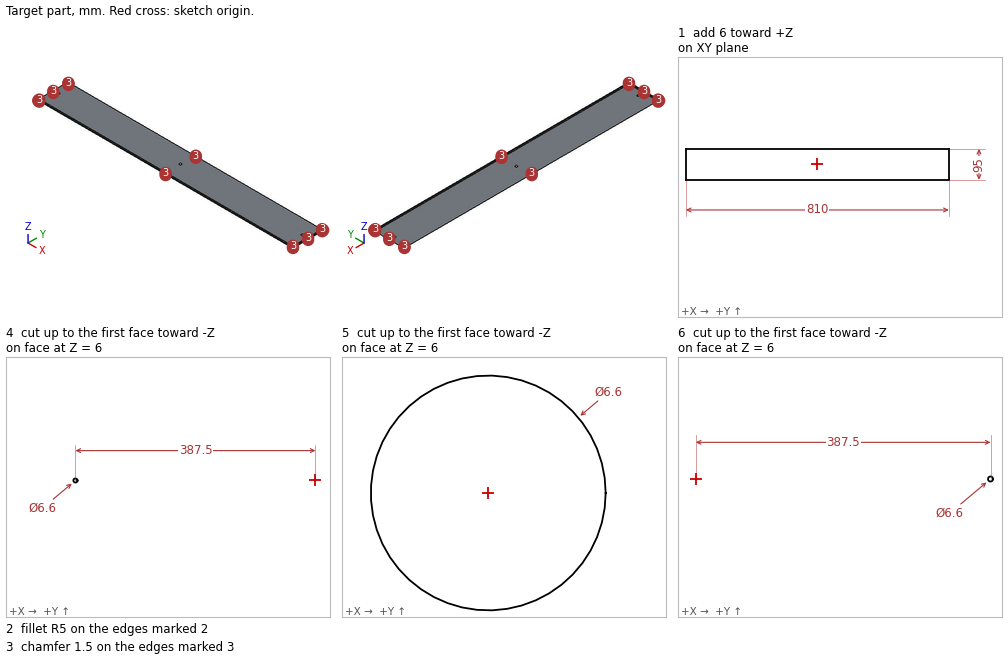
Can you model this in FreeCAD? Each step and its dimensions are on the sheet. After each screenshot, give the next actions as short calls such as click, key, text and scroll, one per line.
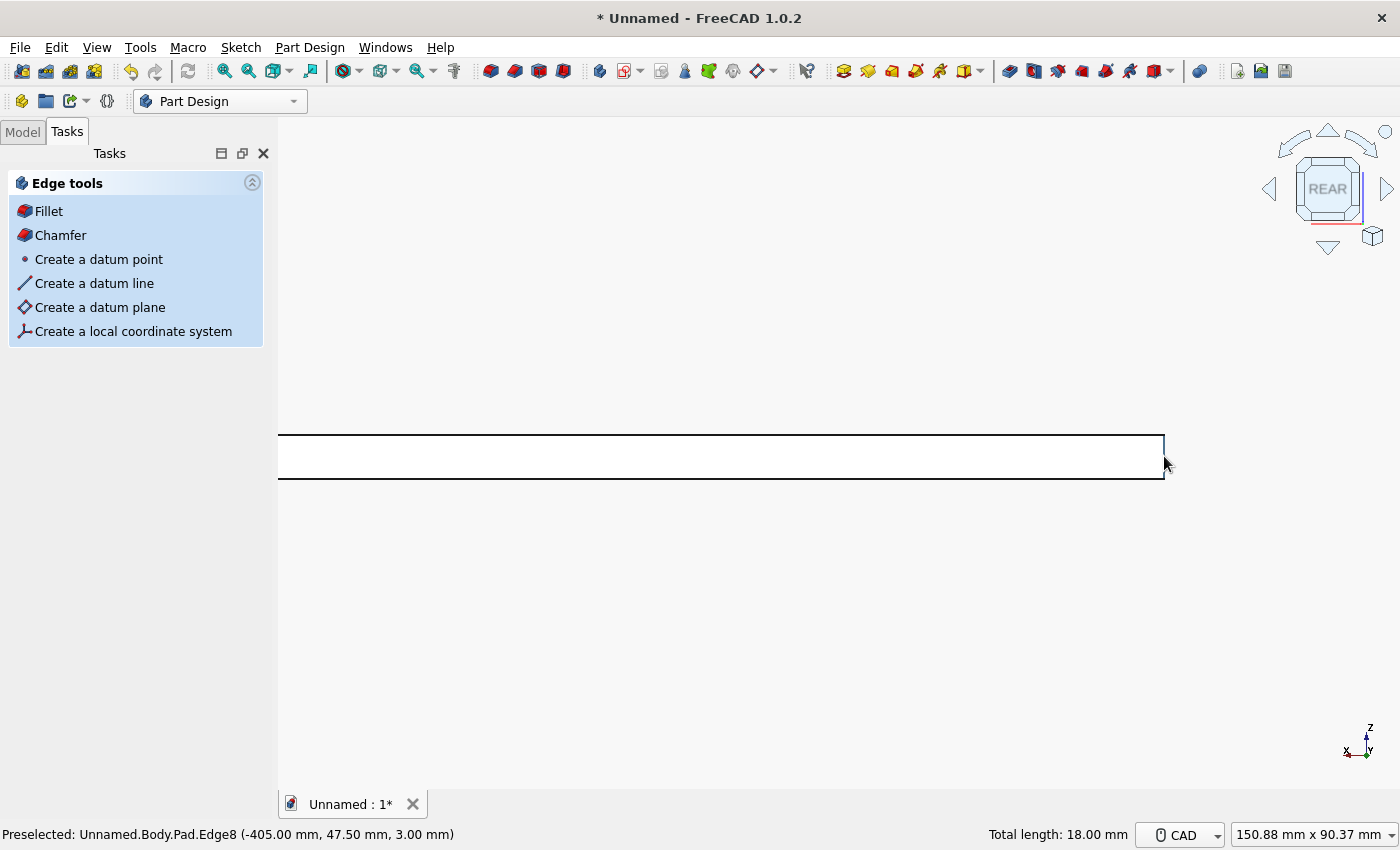
click(226, 72)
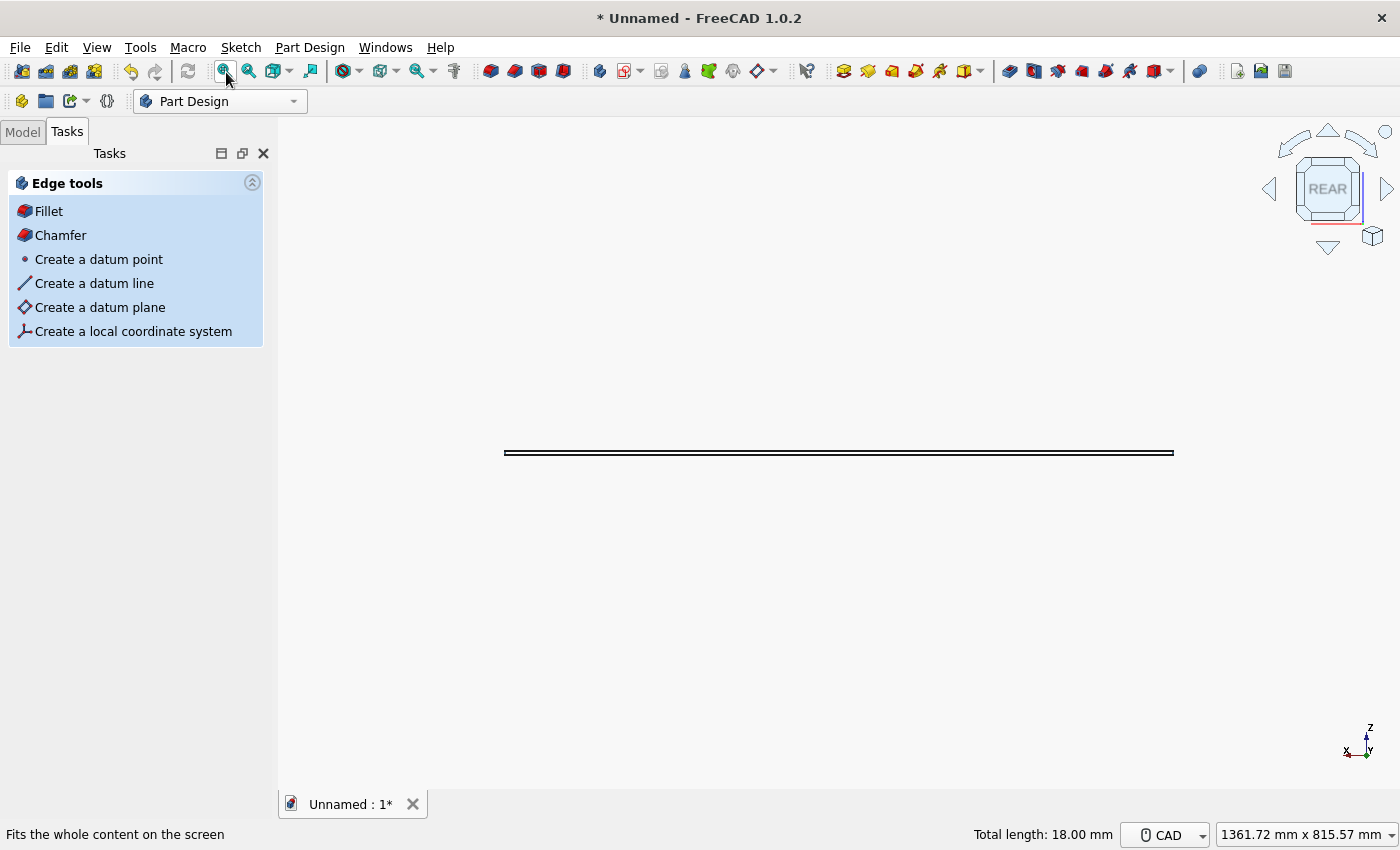
key(6)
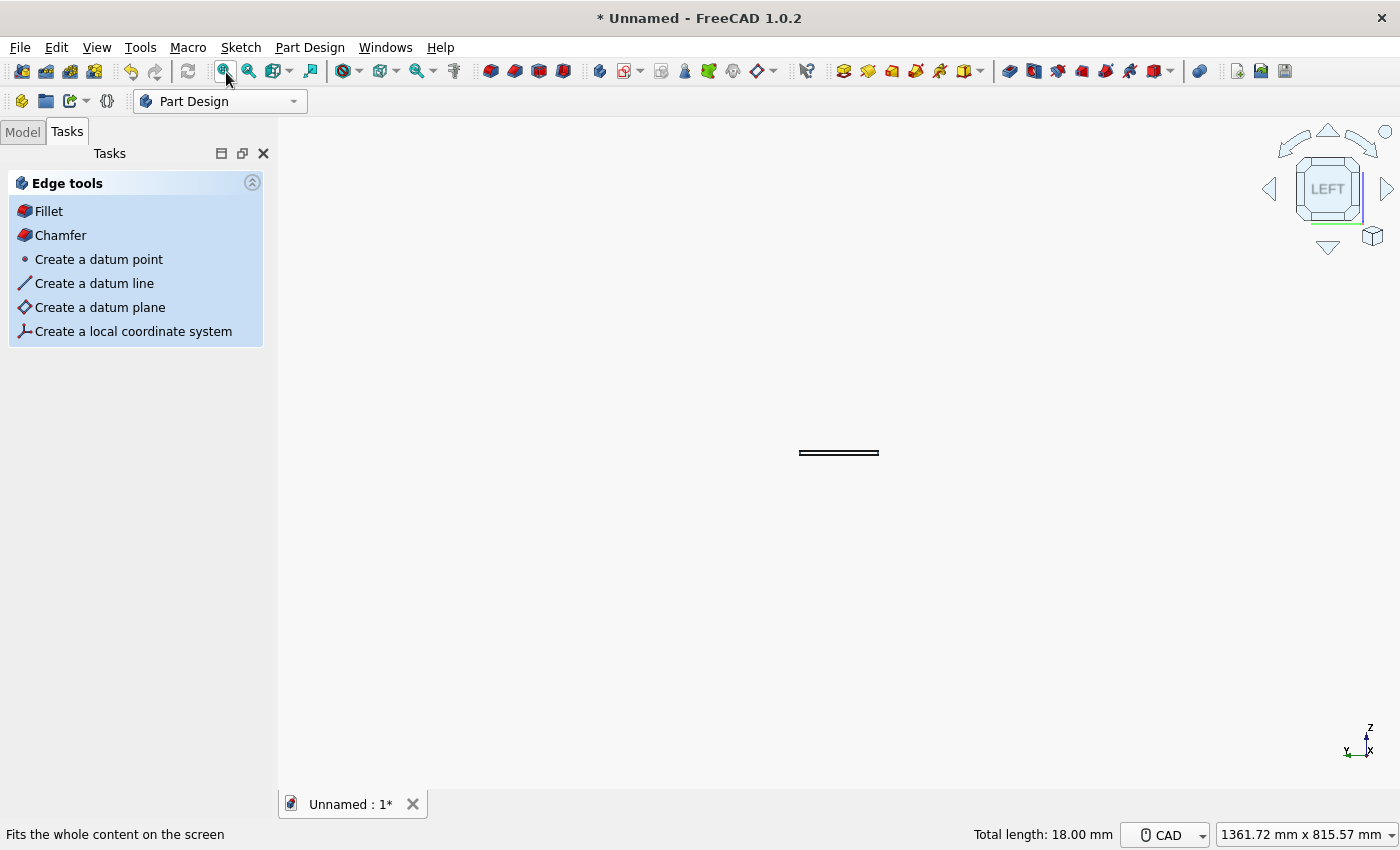
key(v)
key(f)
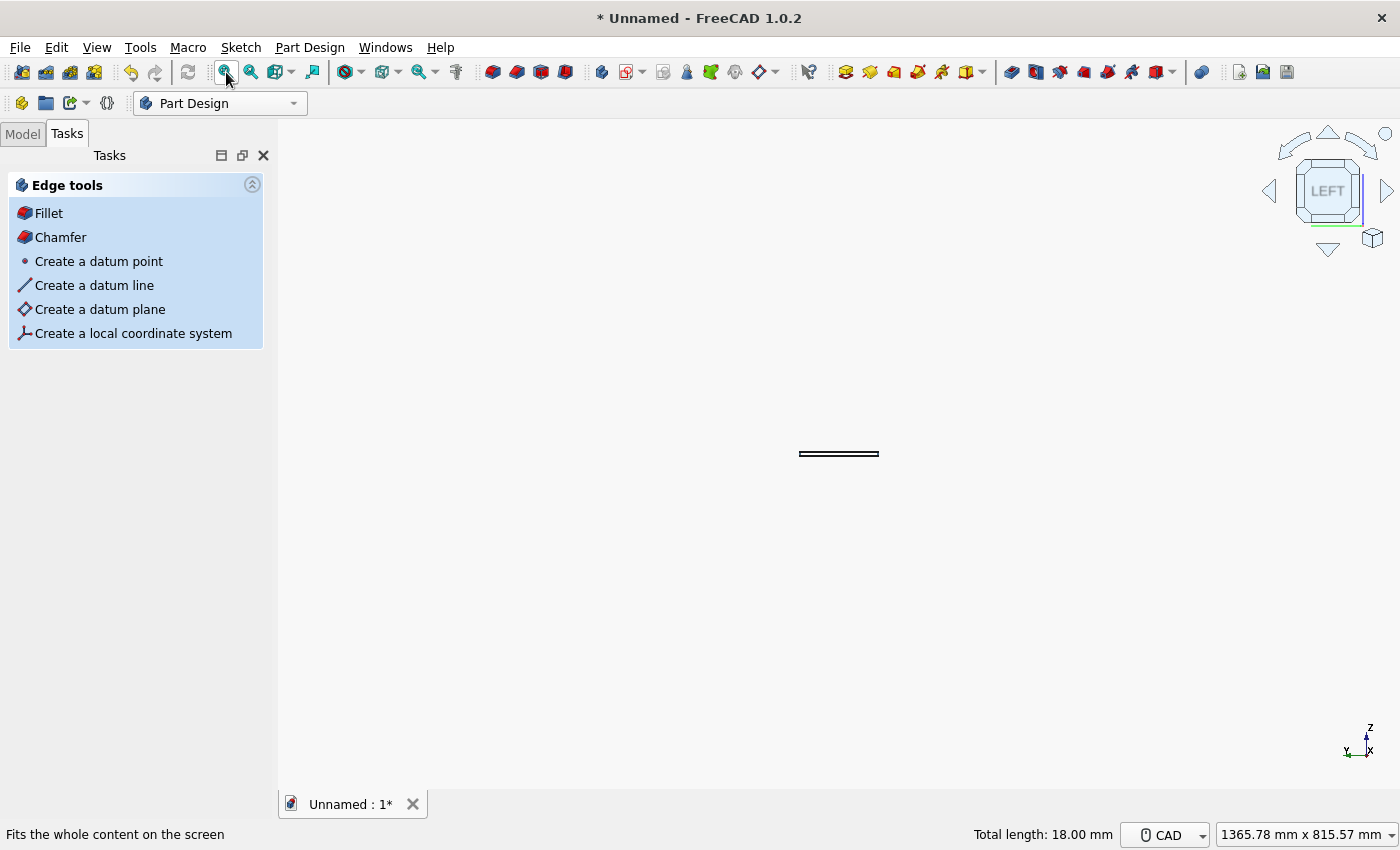
scroll(878, 453, up, 11)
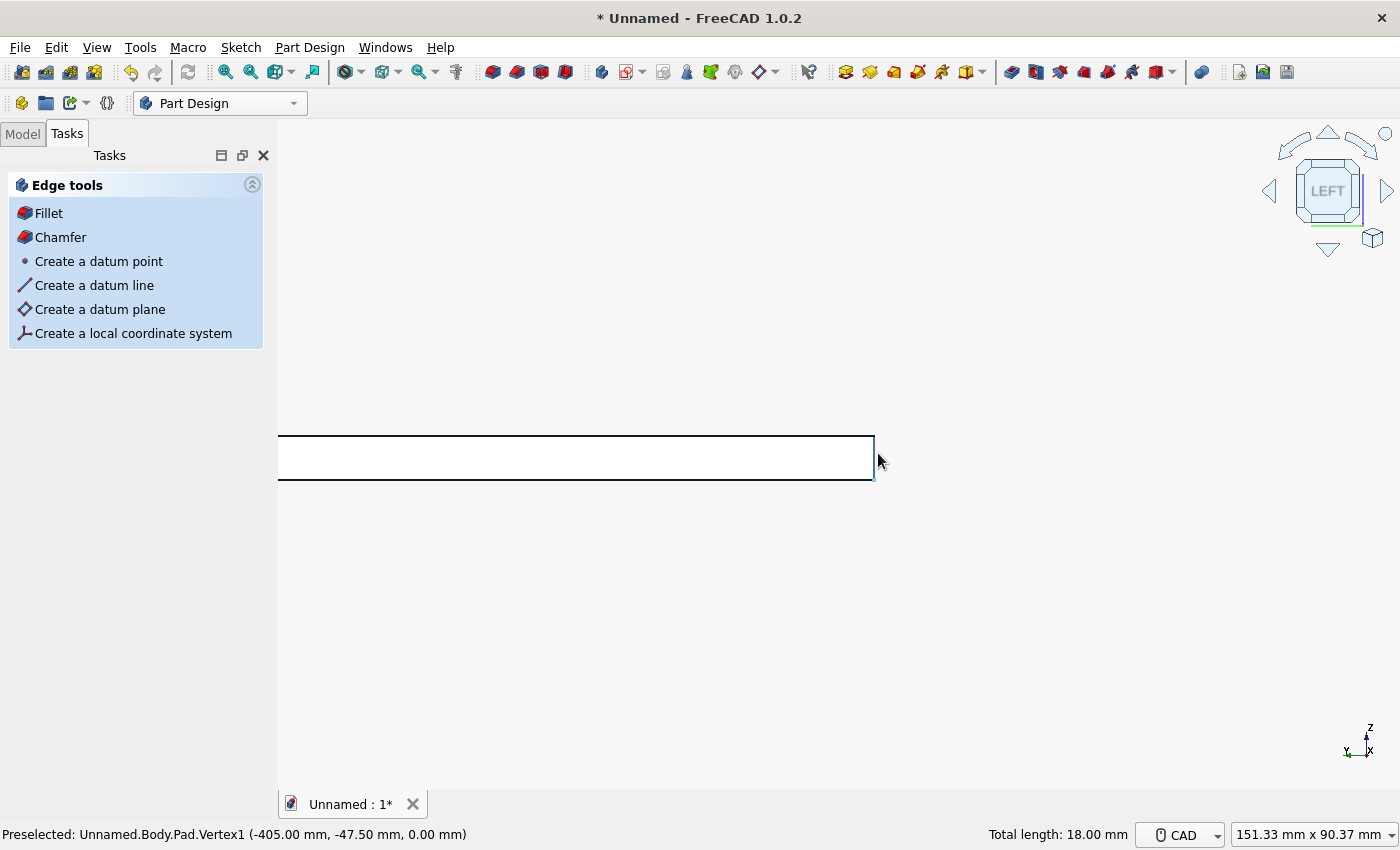
click(226, 72)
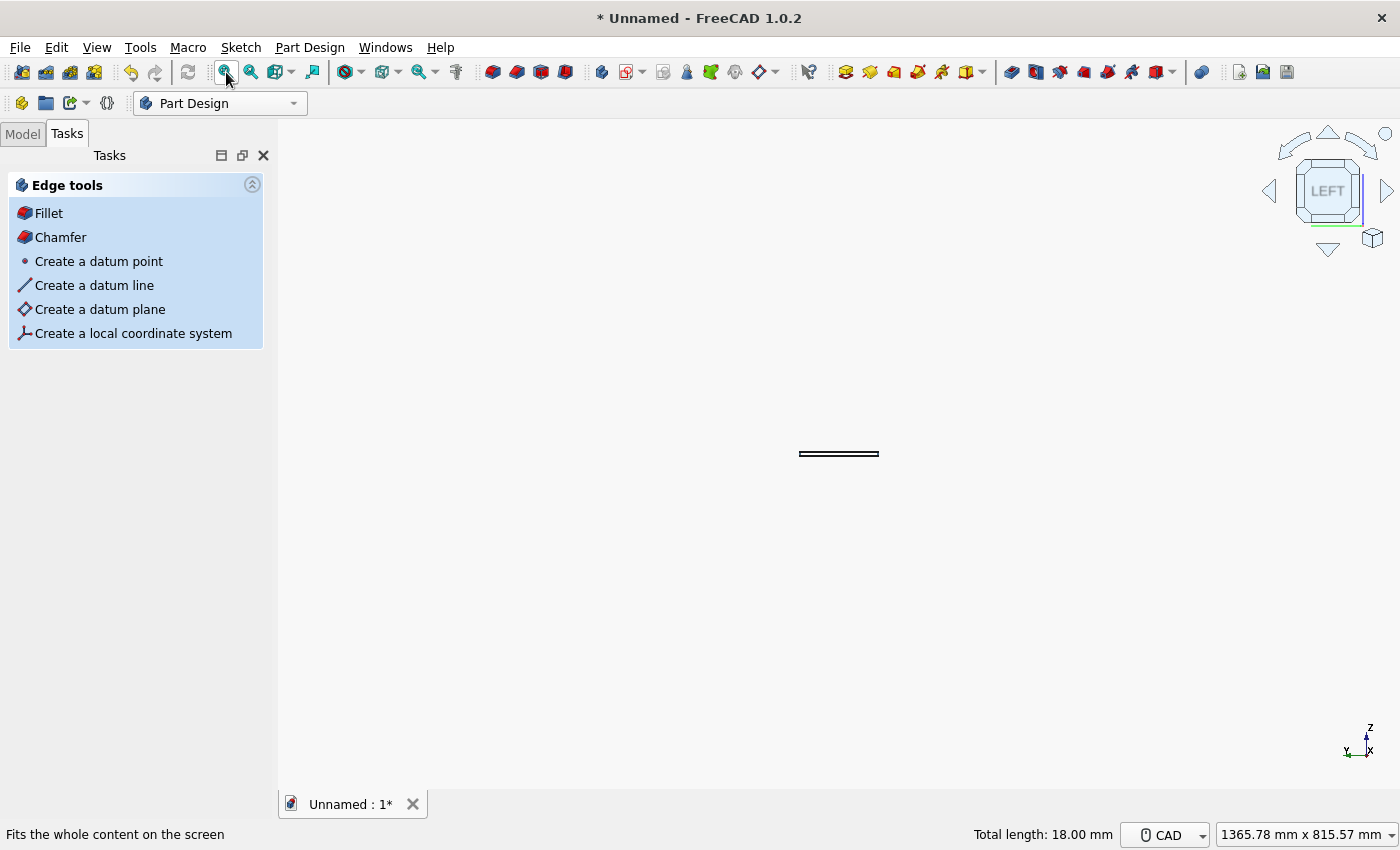
key(v)
key(3)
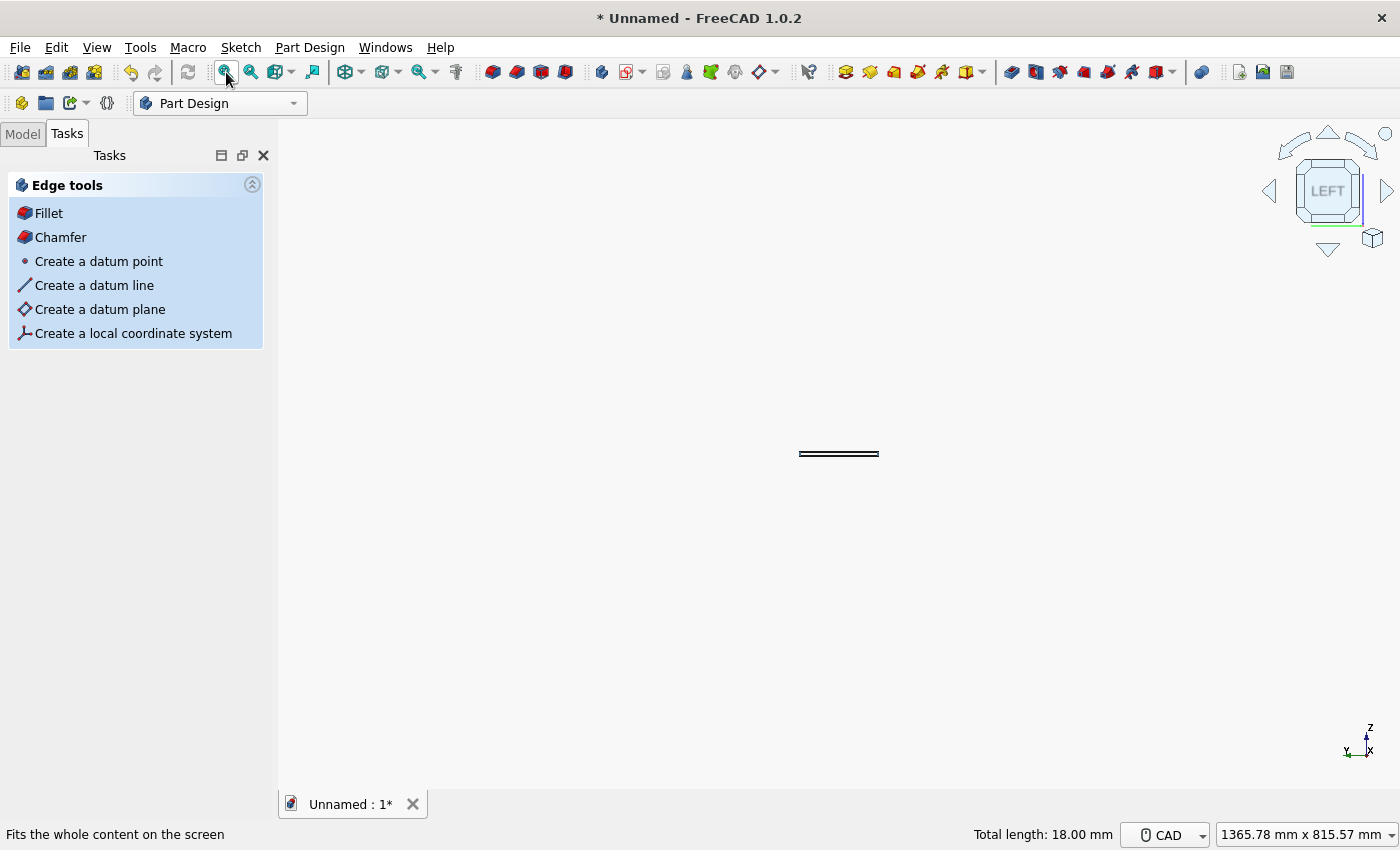
key(0)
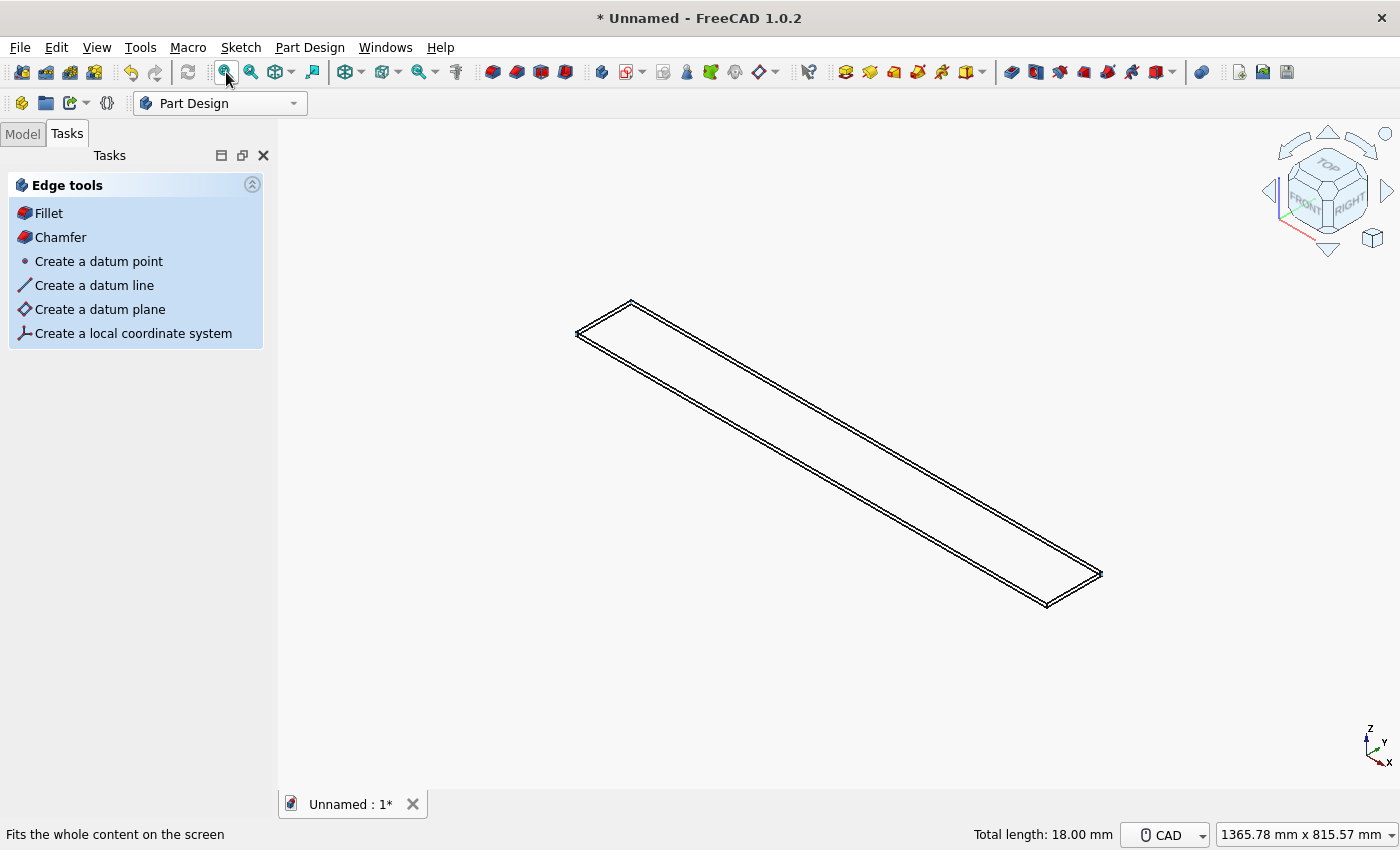
scroll(1047, 605, up, 11)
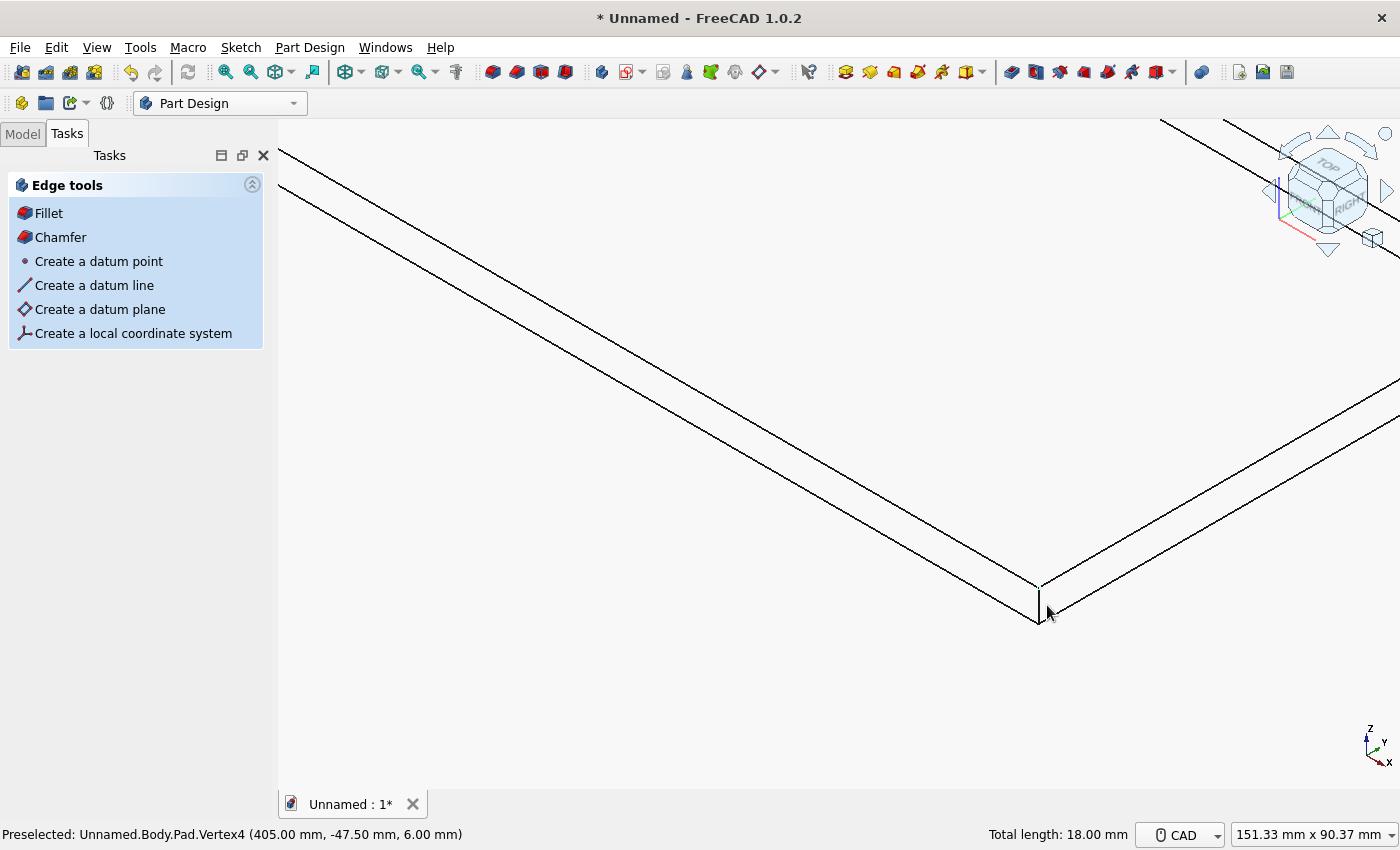
click(1039, 605, ctrl)